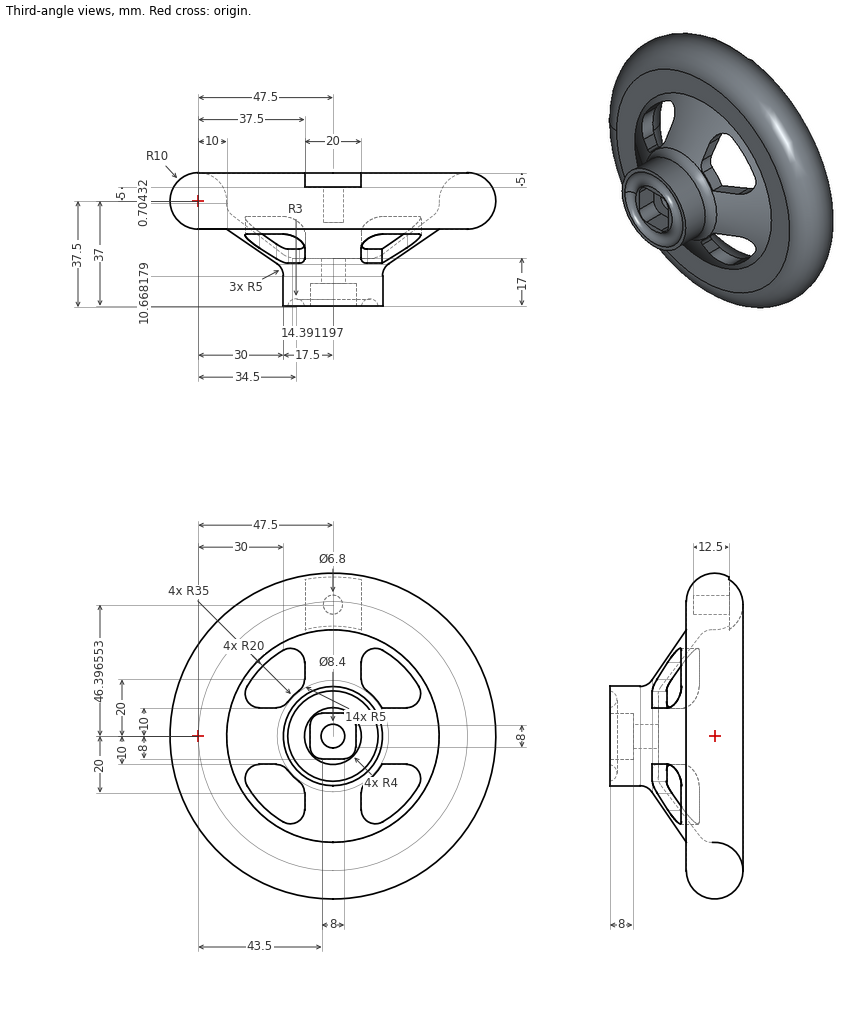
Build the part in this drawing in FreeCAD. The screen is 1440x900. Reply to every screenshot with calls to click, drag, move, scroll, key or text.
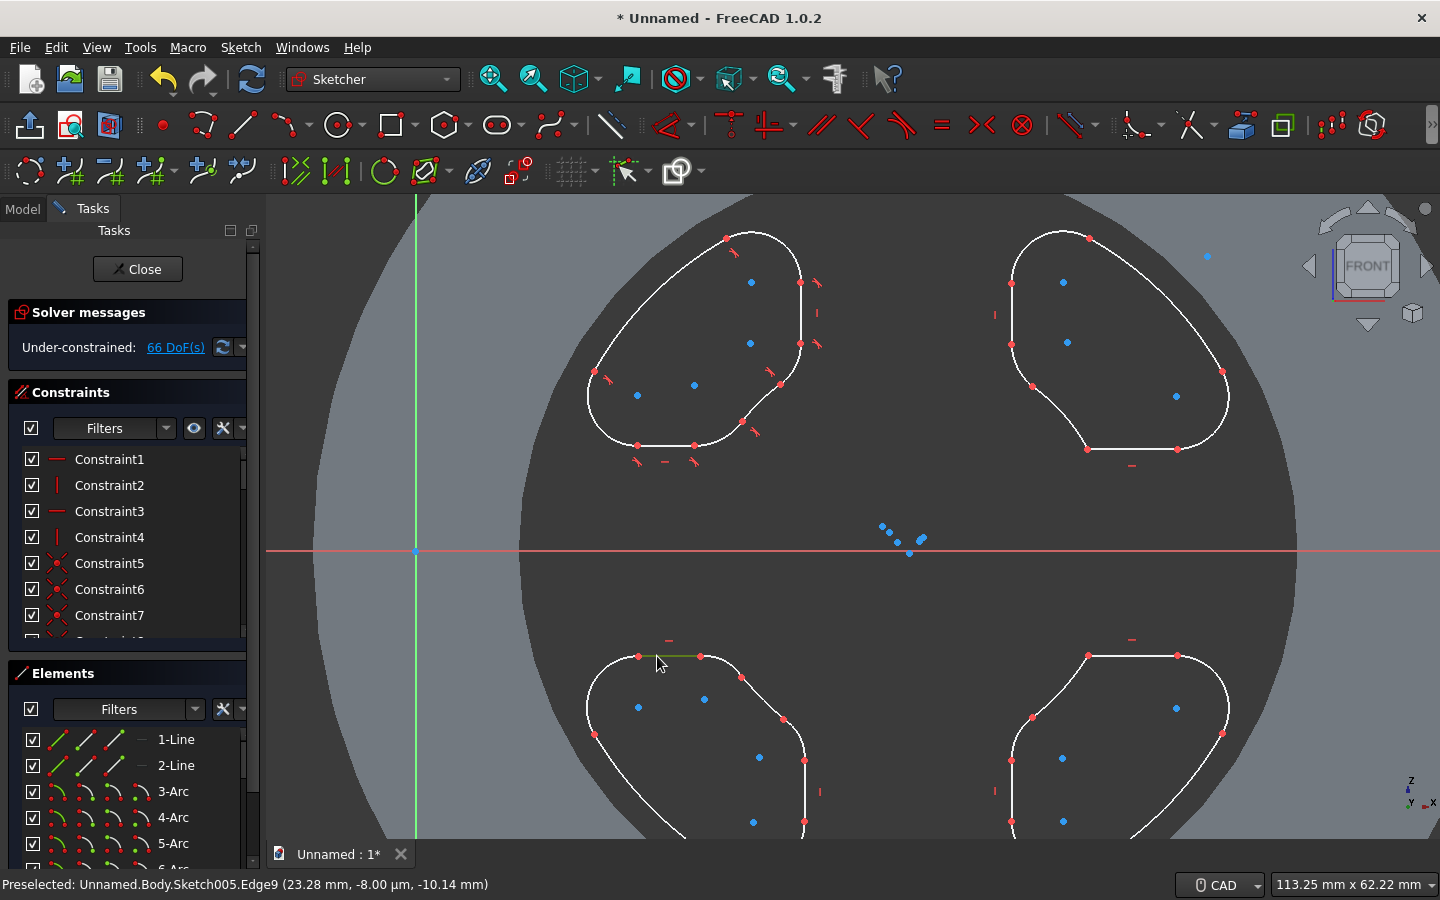
click(732, 666)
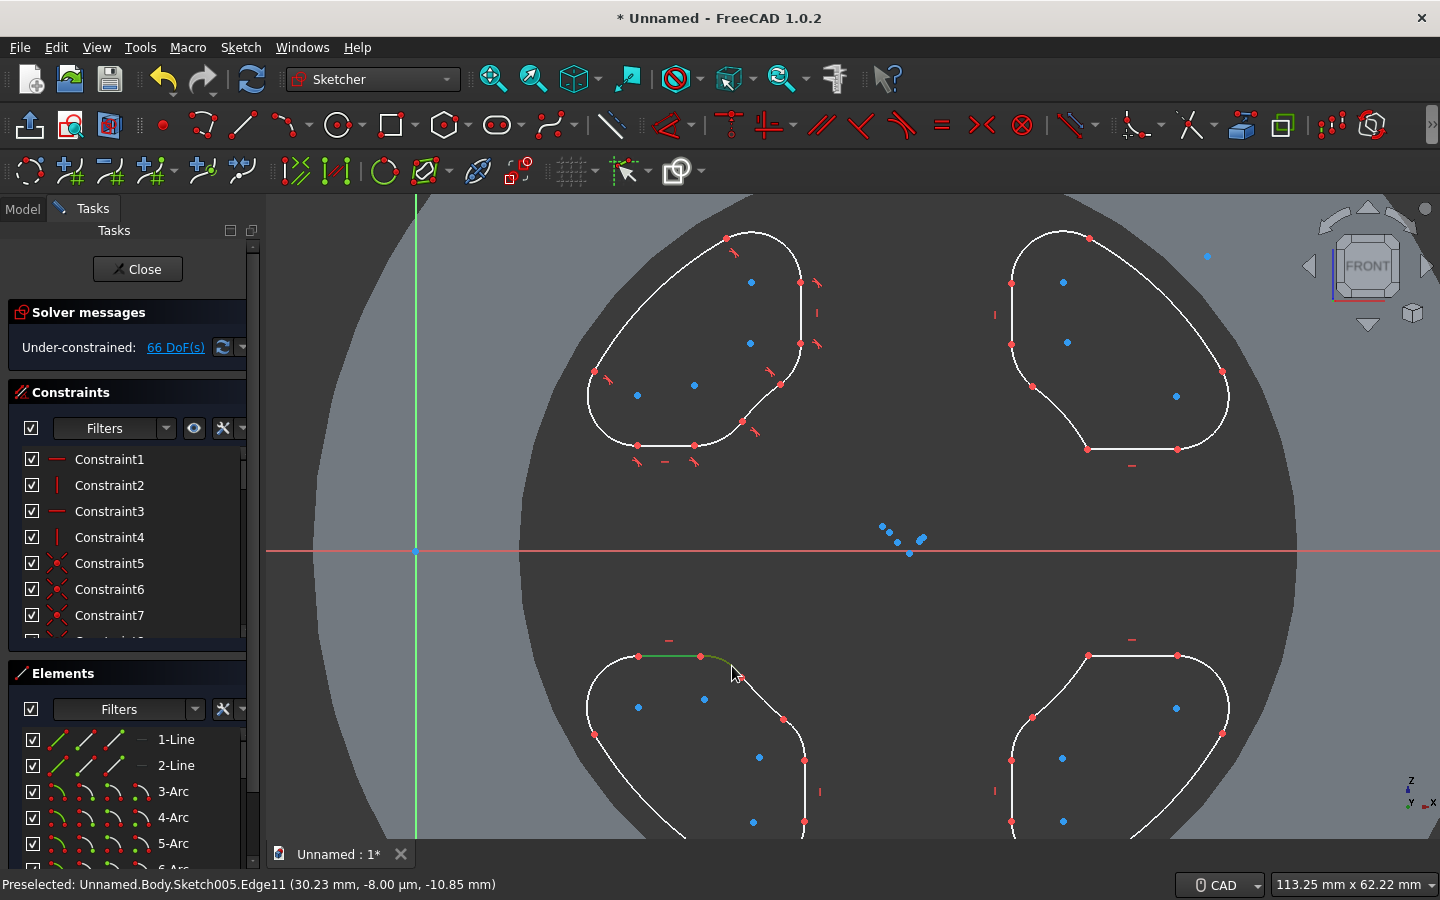
click(902, 126)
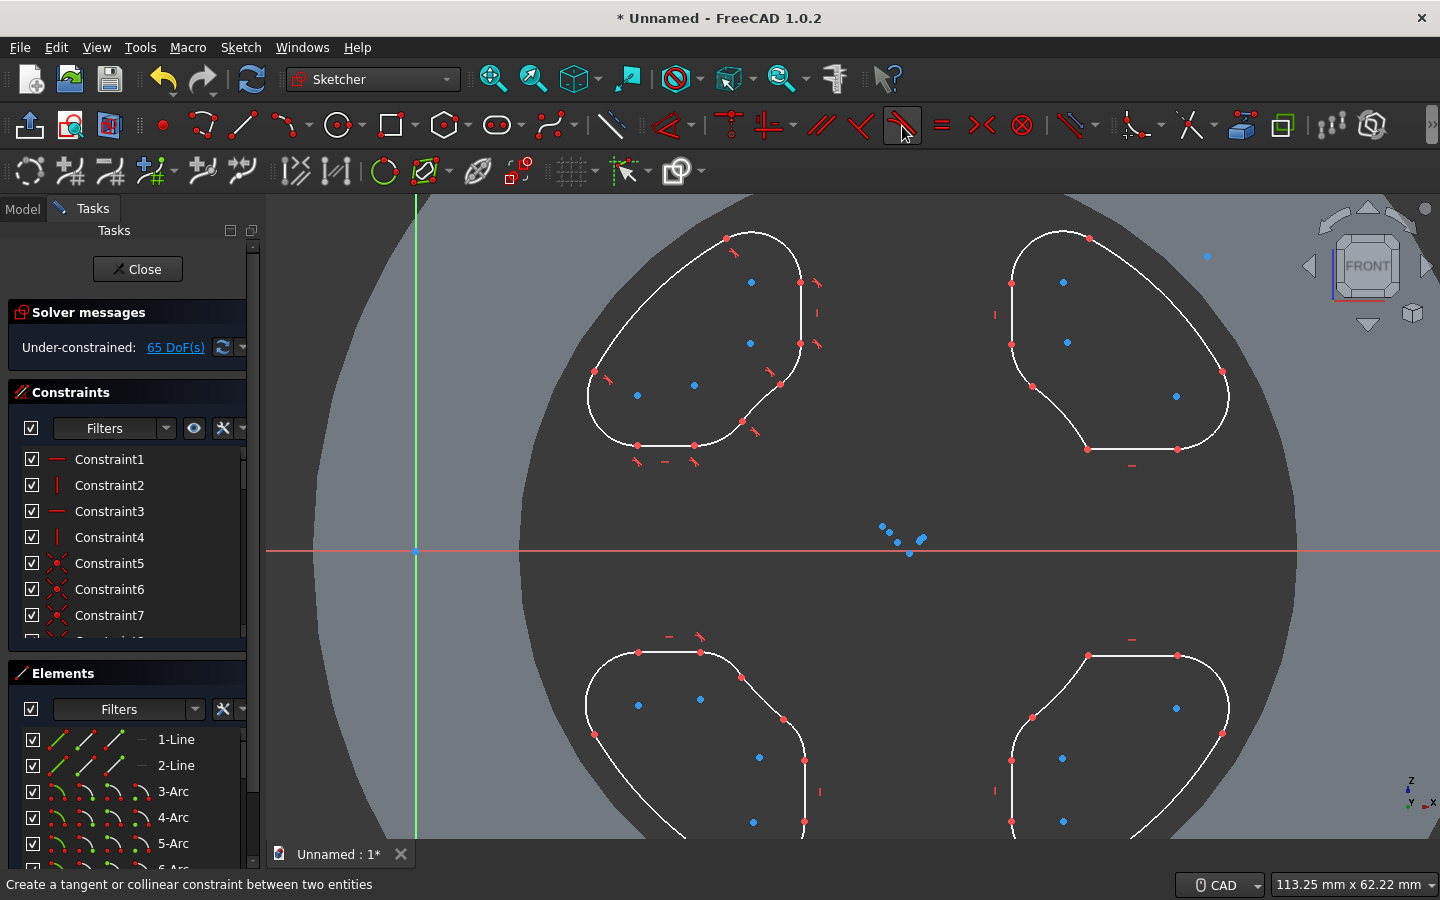
click(657, 652)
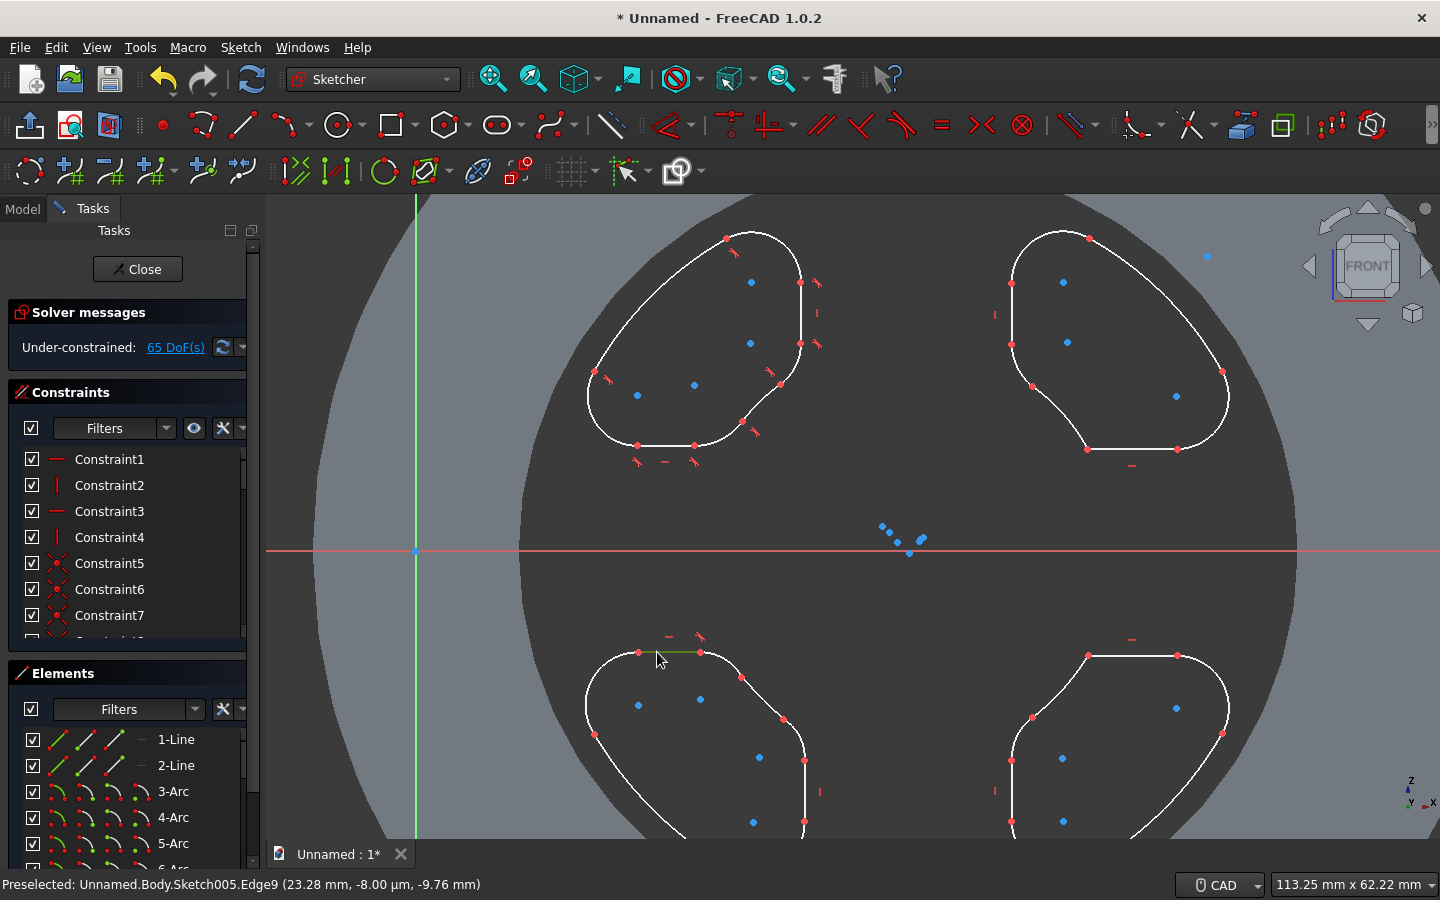
click(607, 663)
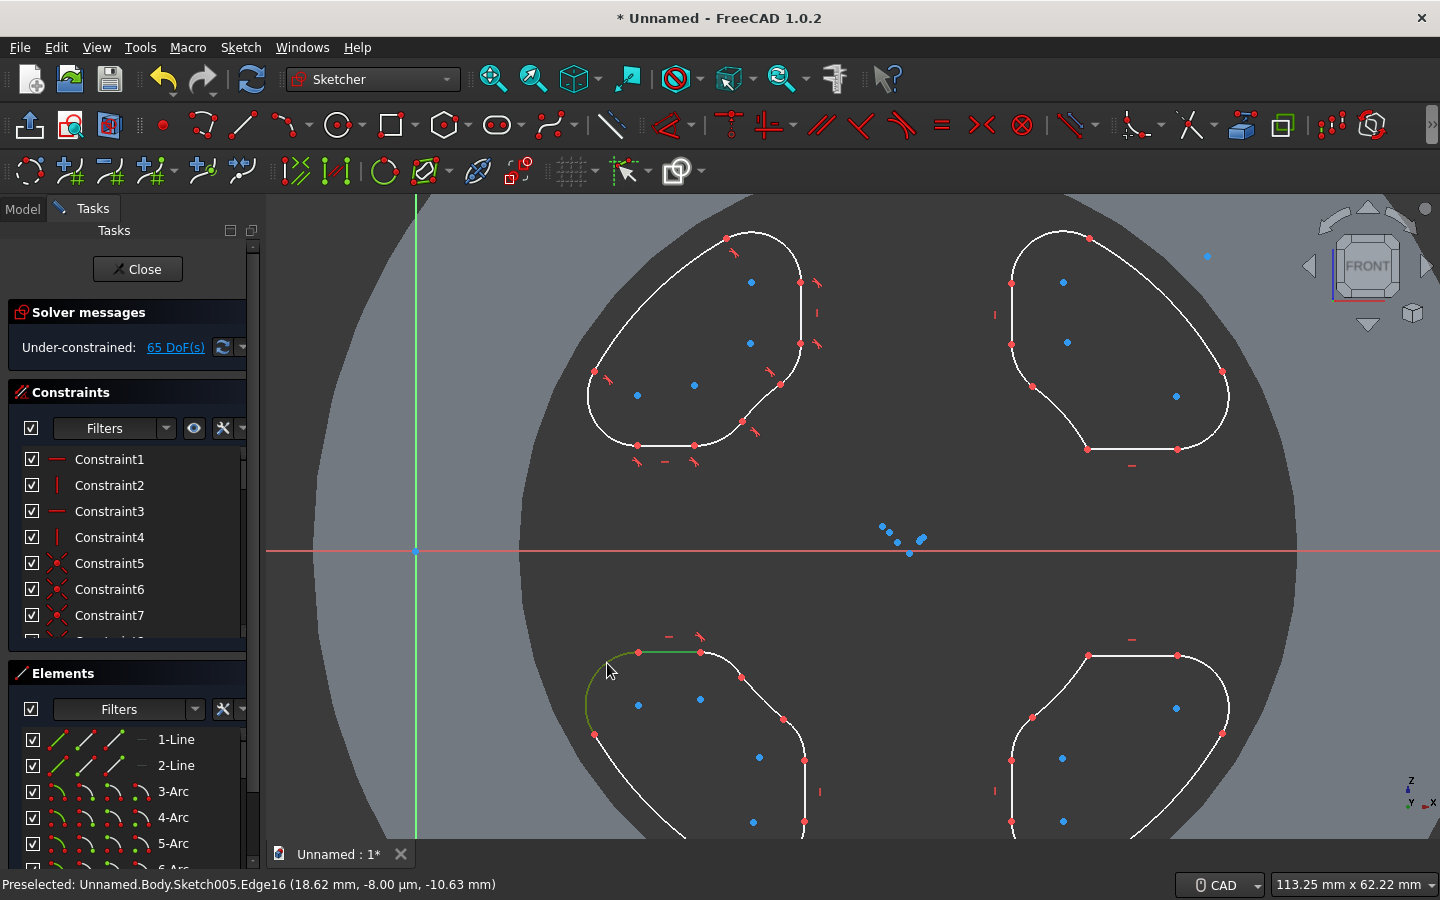
click(902, 126)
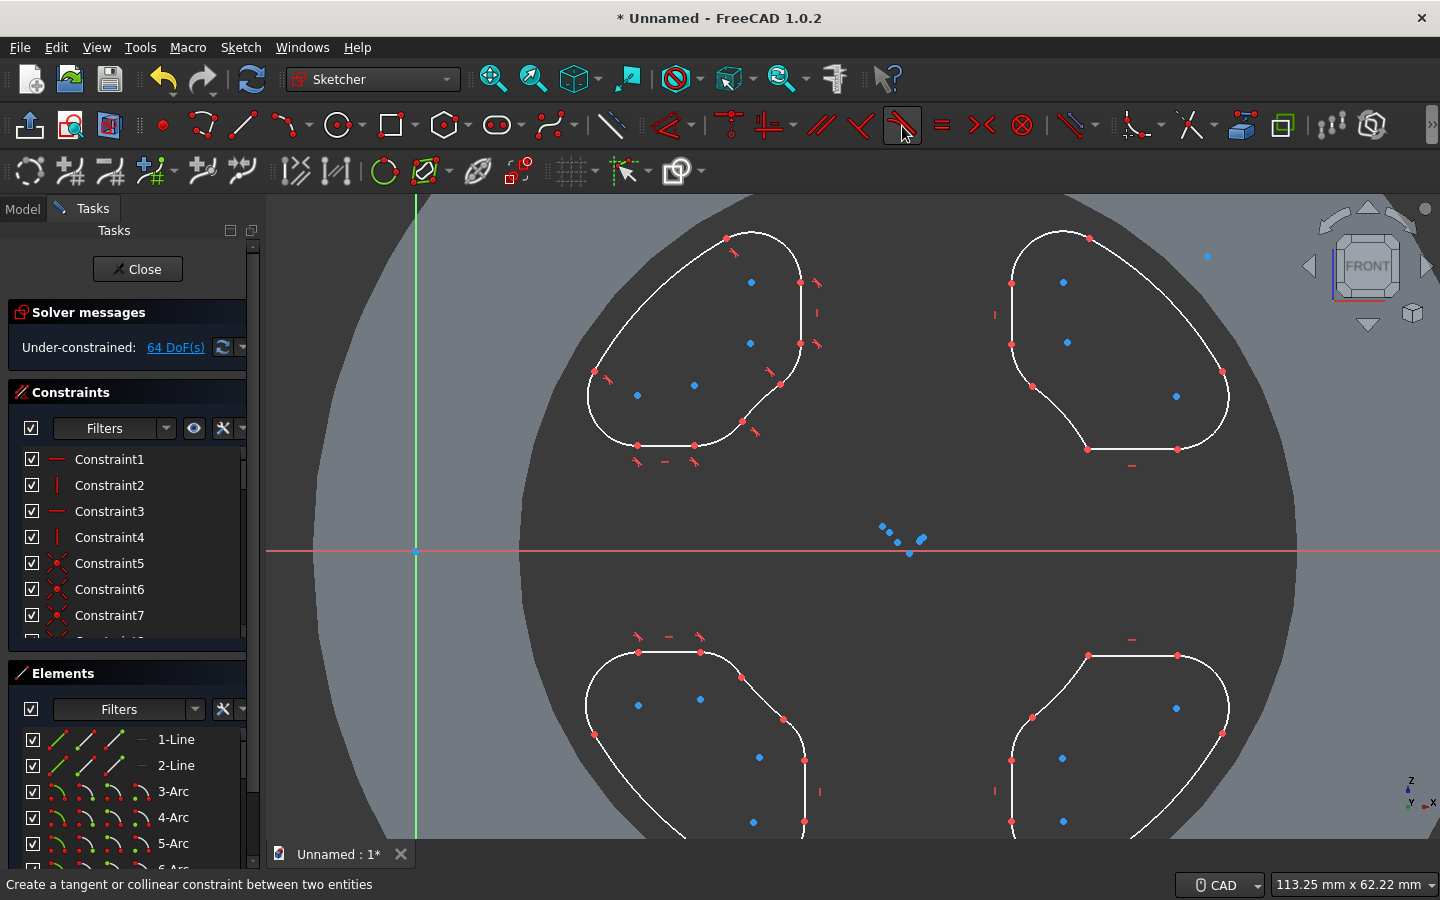
click(805, 779)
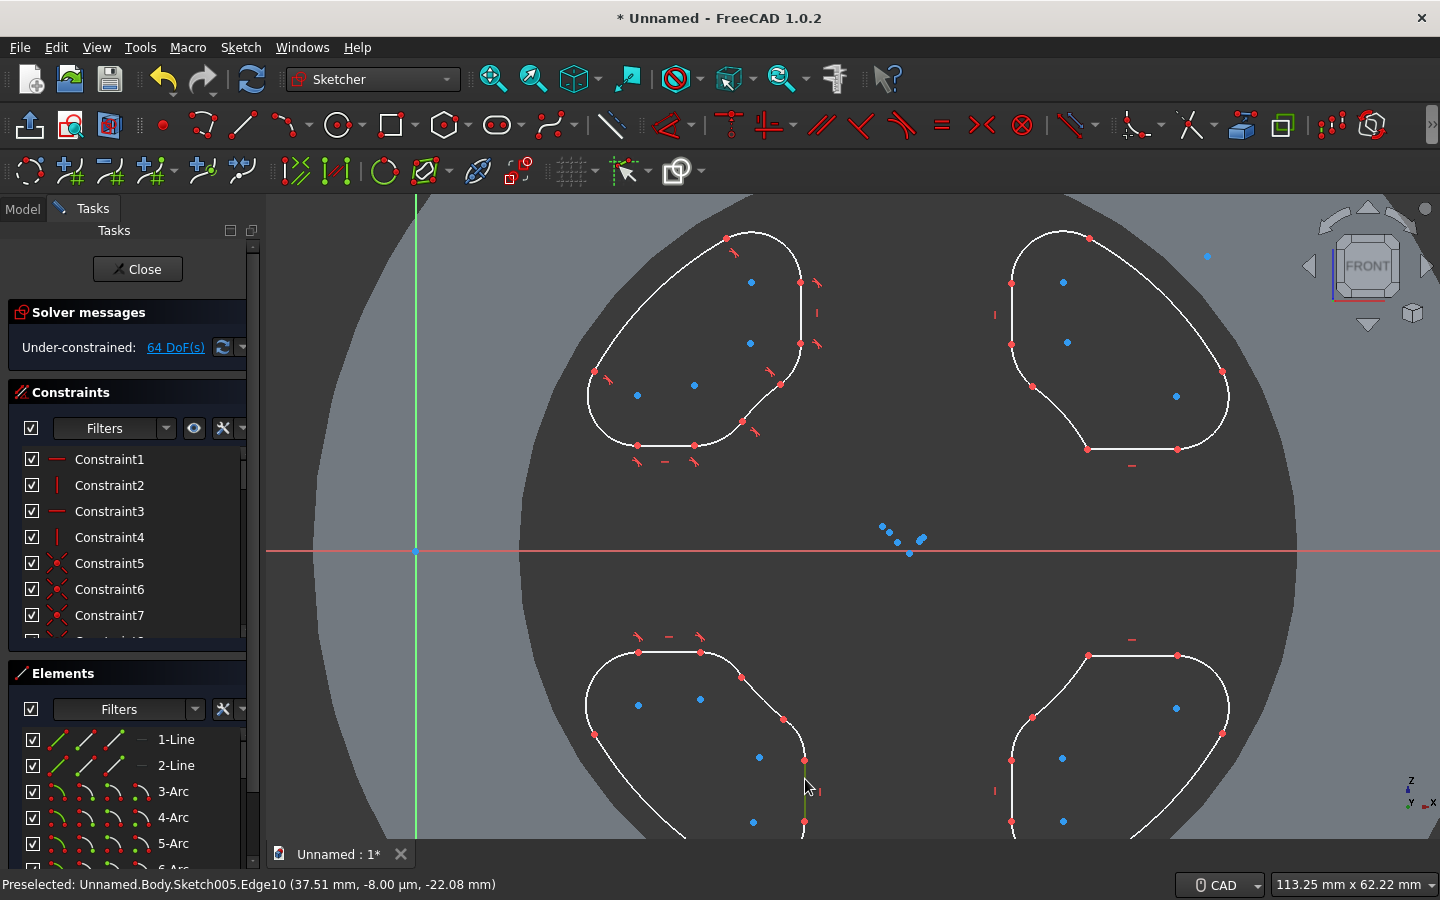
click(803, 746)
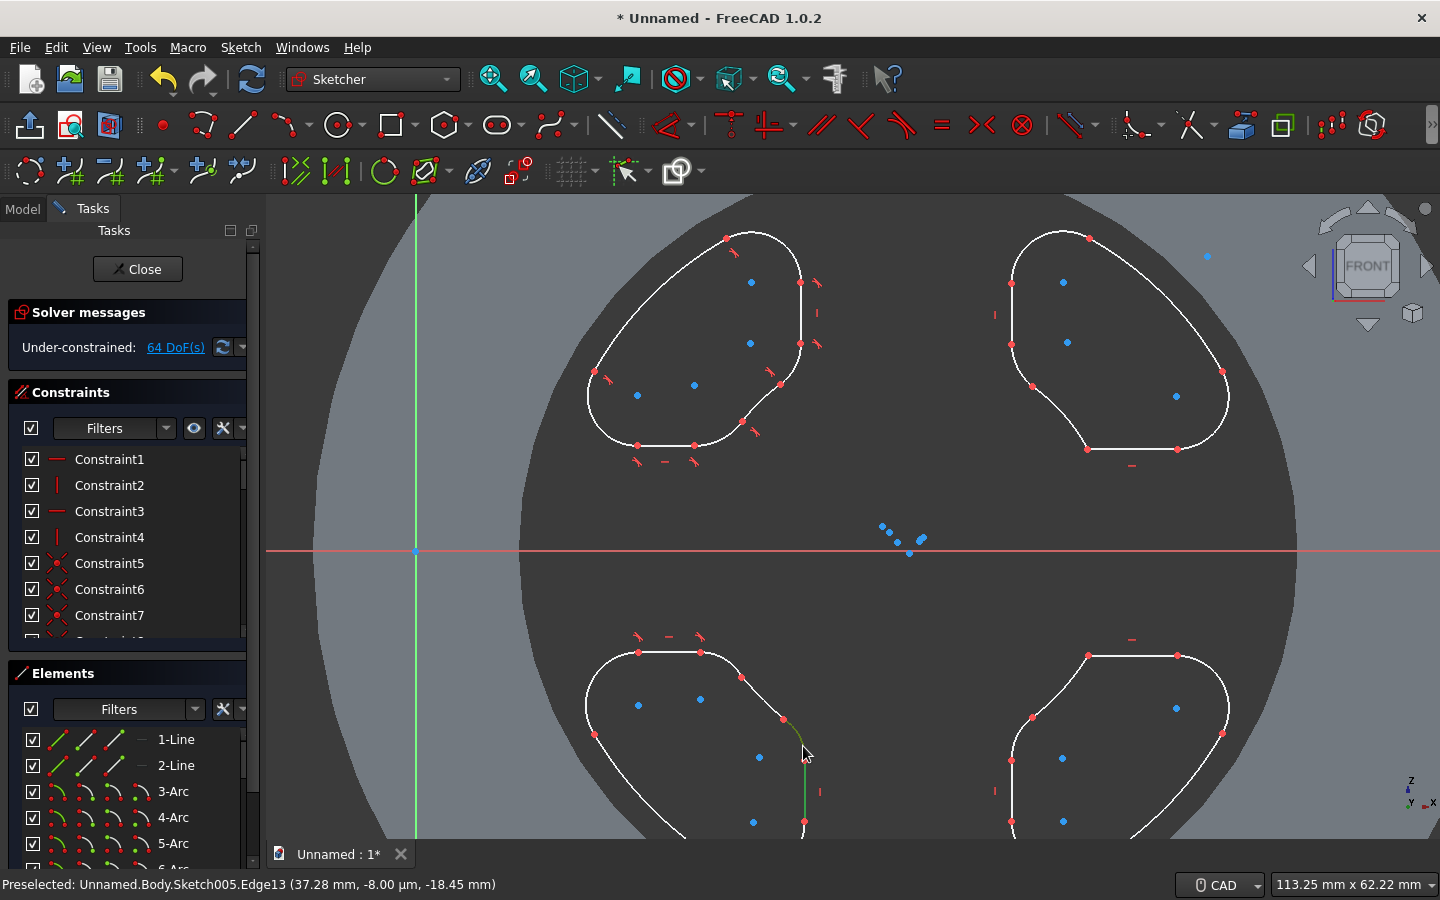
click(902, 126)